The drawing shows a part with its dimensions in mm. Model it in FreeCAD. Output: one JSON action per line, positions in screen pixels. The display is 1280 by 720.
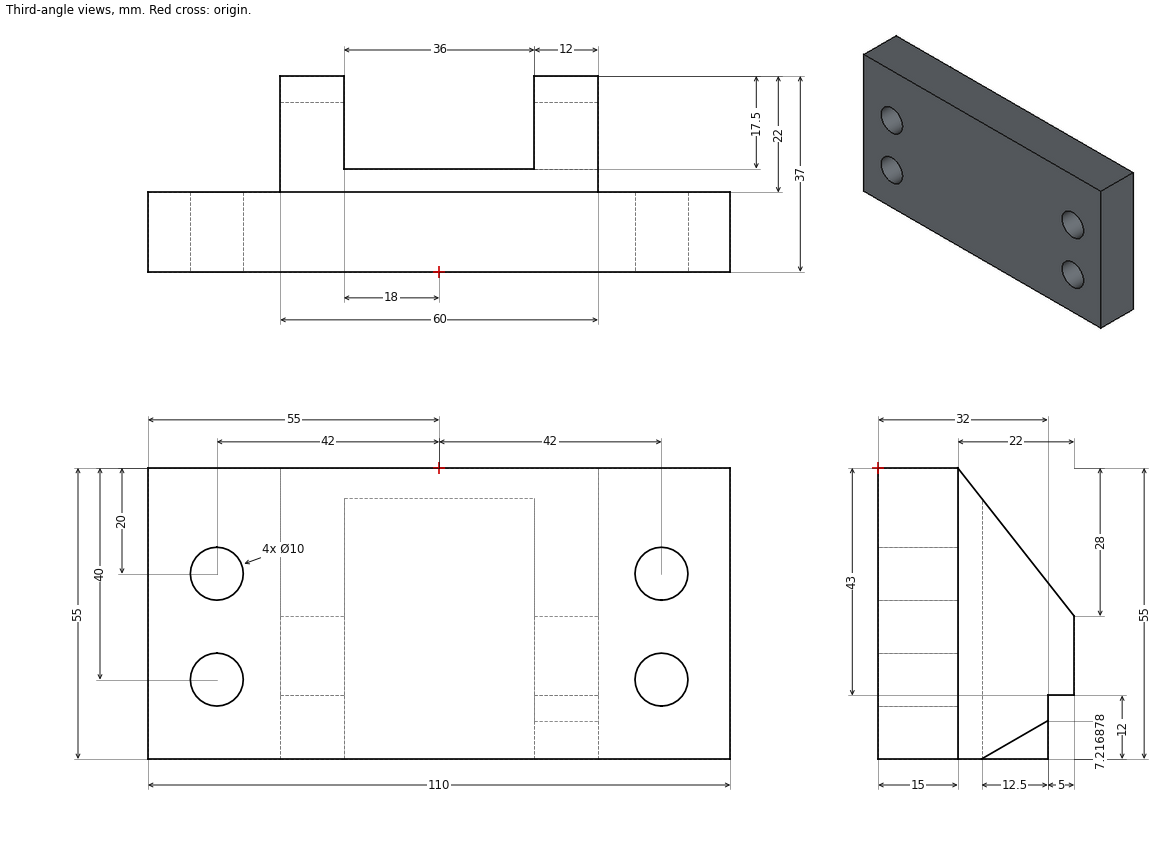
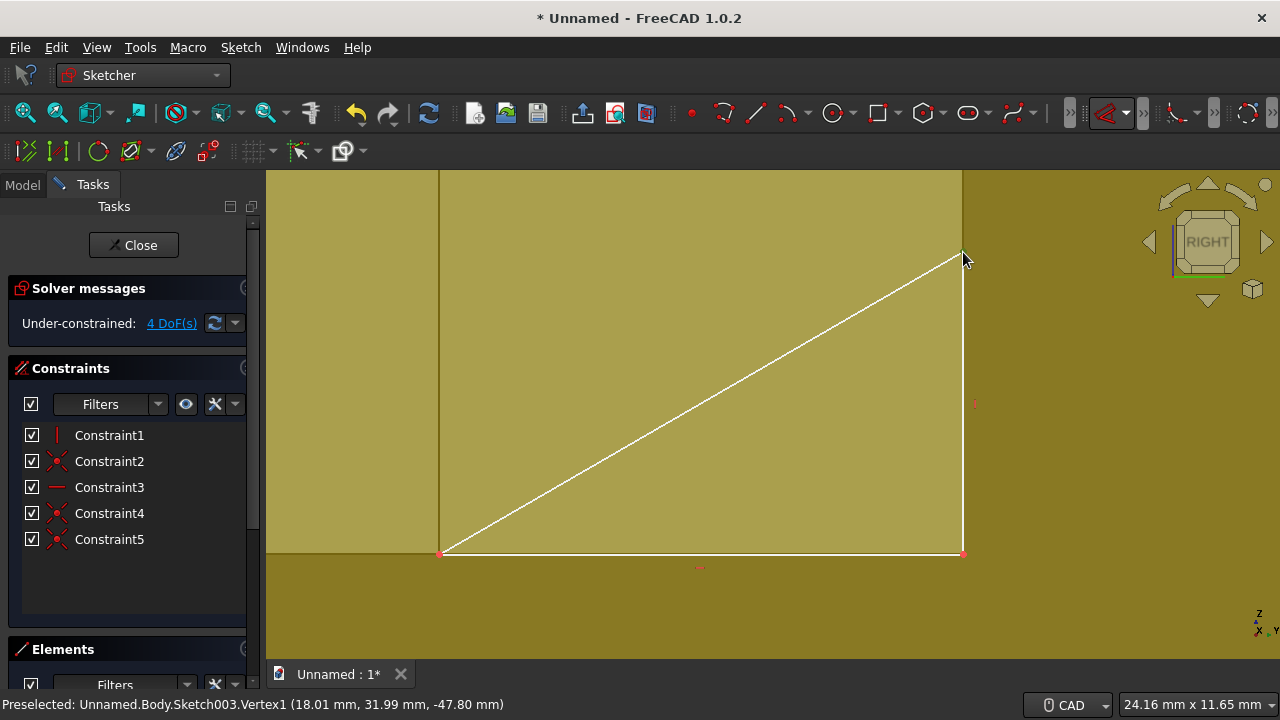
{"action": "key", "text": "l"}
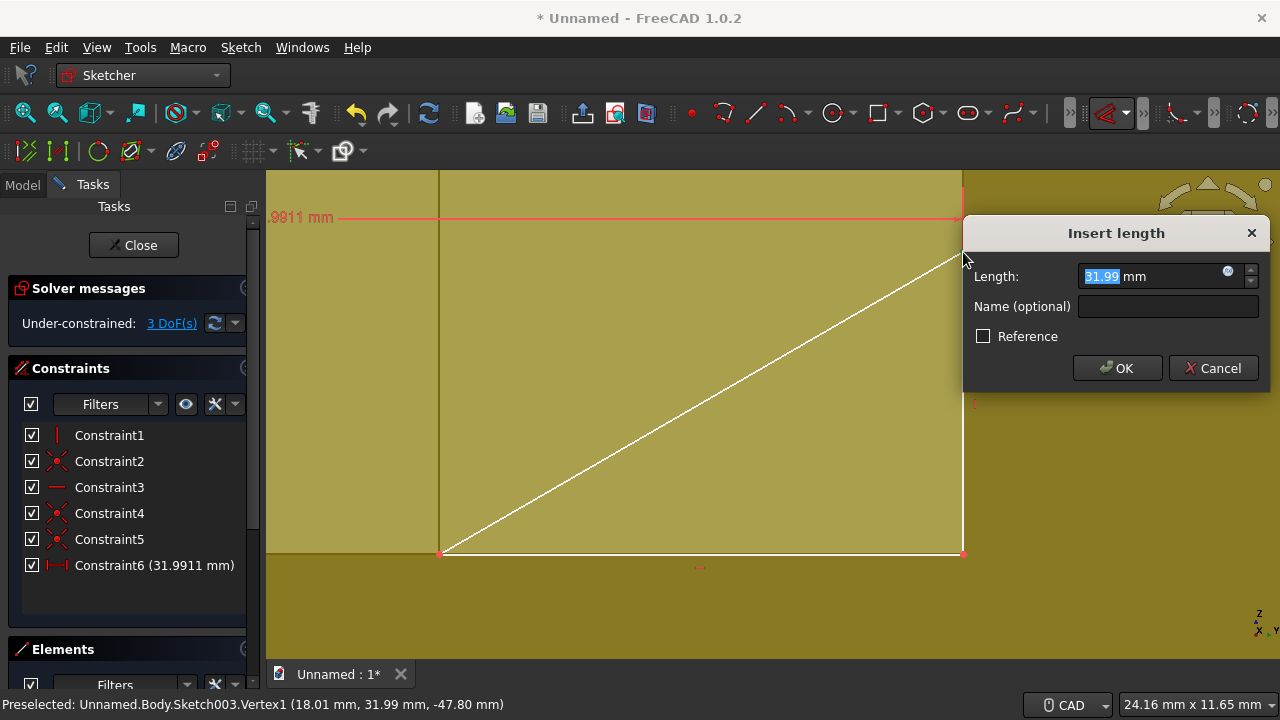
{"action": "type", "text": "32"}
{"action": "key", "text": "Return"}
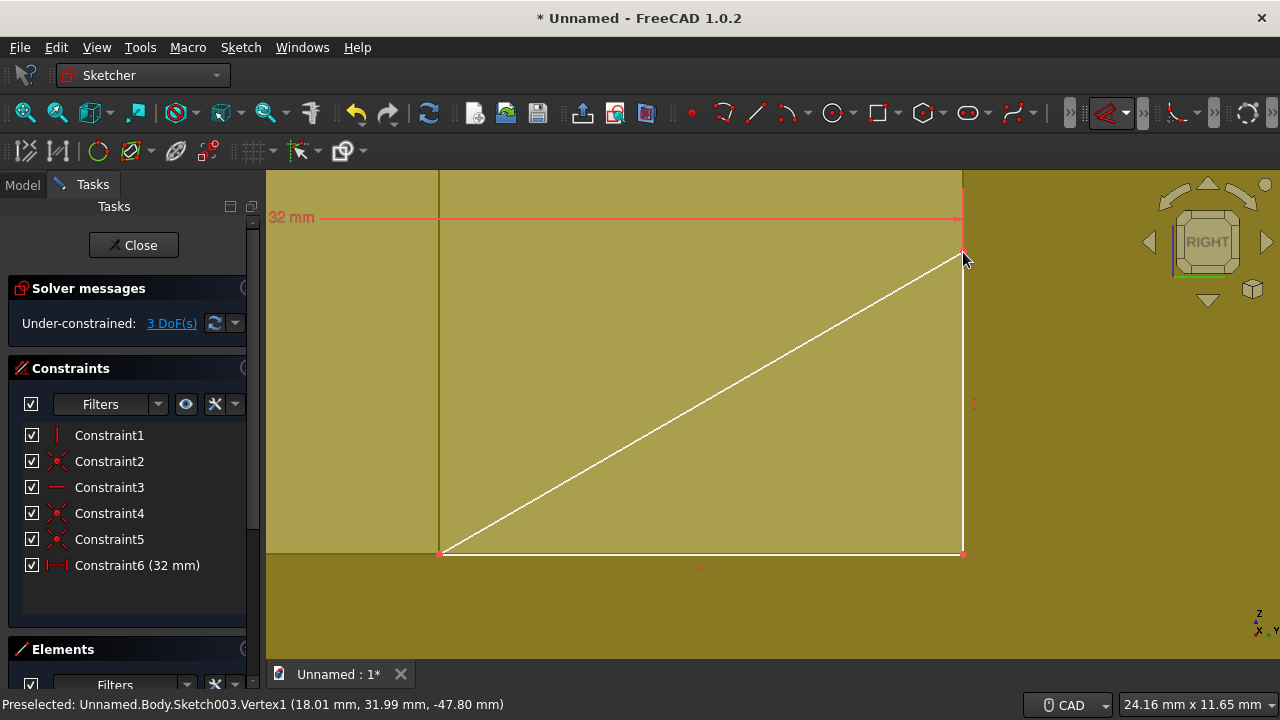
{"action": "left_click", "coordinate": [963, 555]}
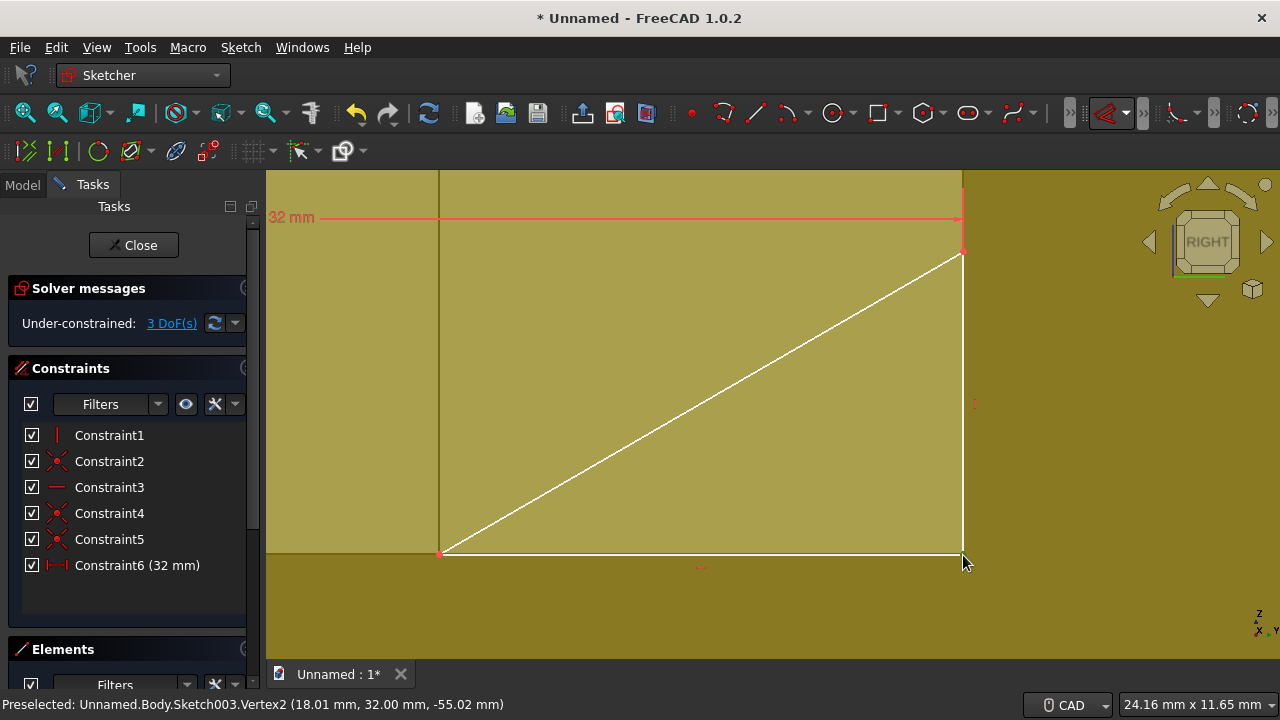
{"action": "key", "text": "i"}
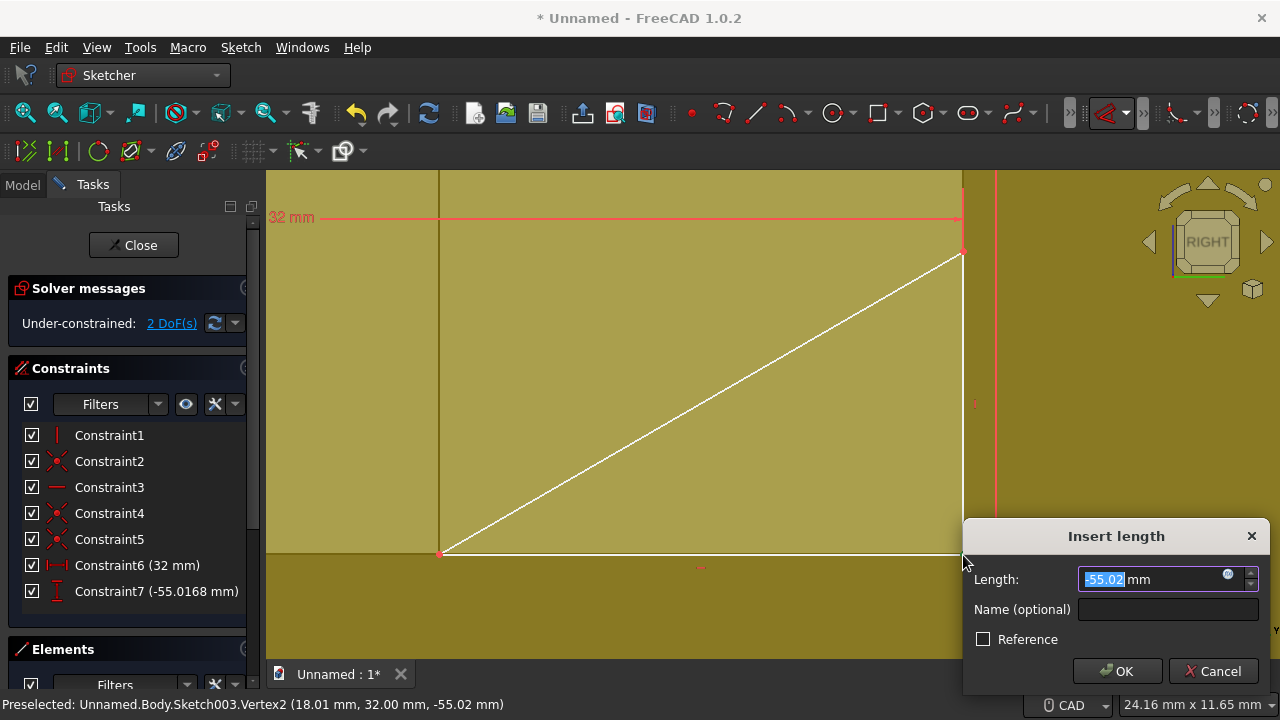
{"action": "type", "text": "-55"}
{"action": "key", "text": "Return"}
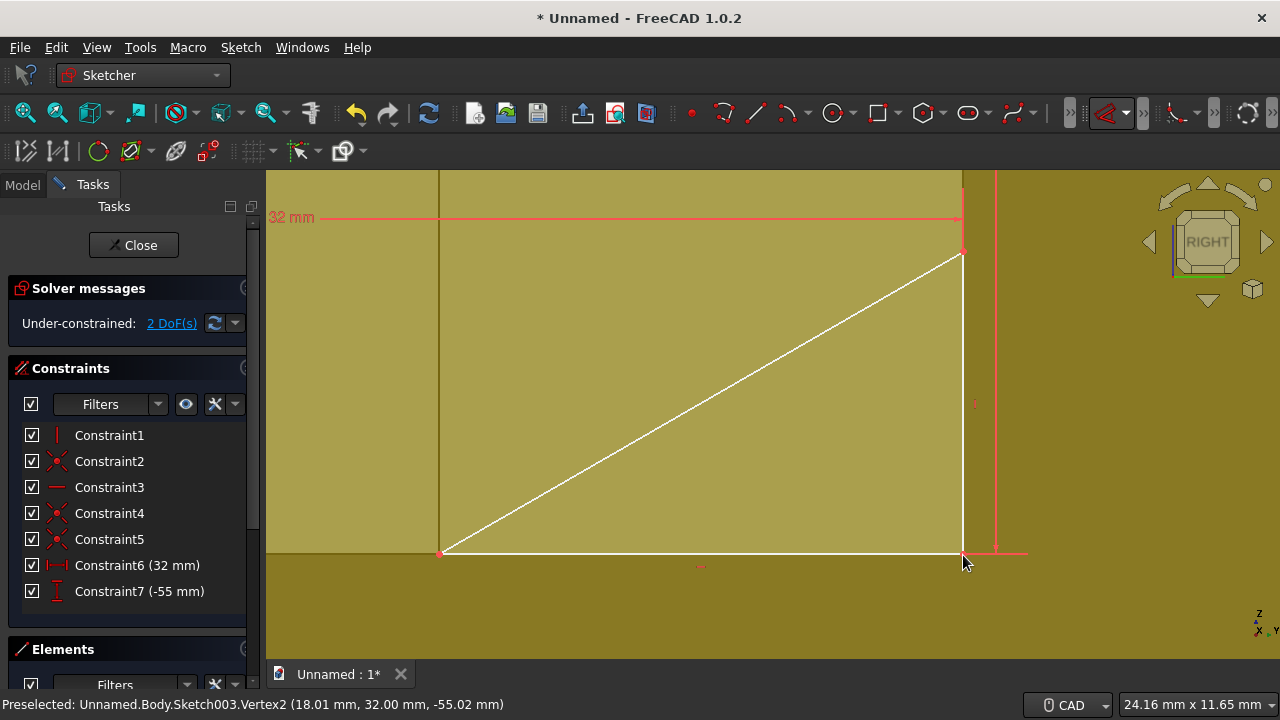
{"action": "left_click", "coordinate": [806, 554]}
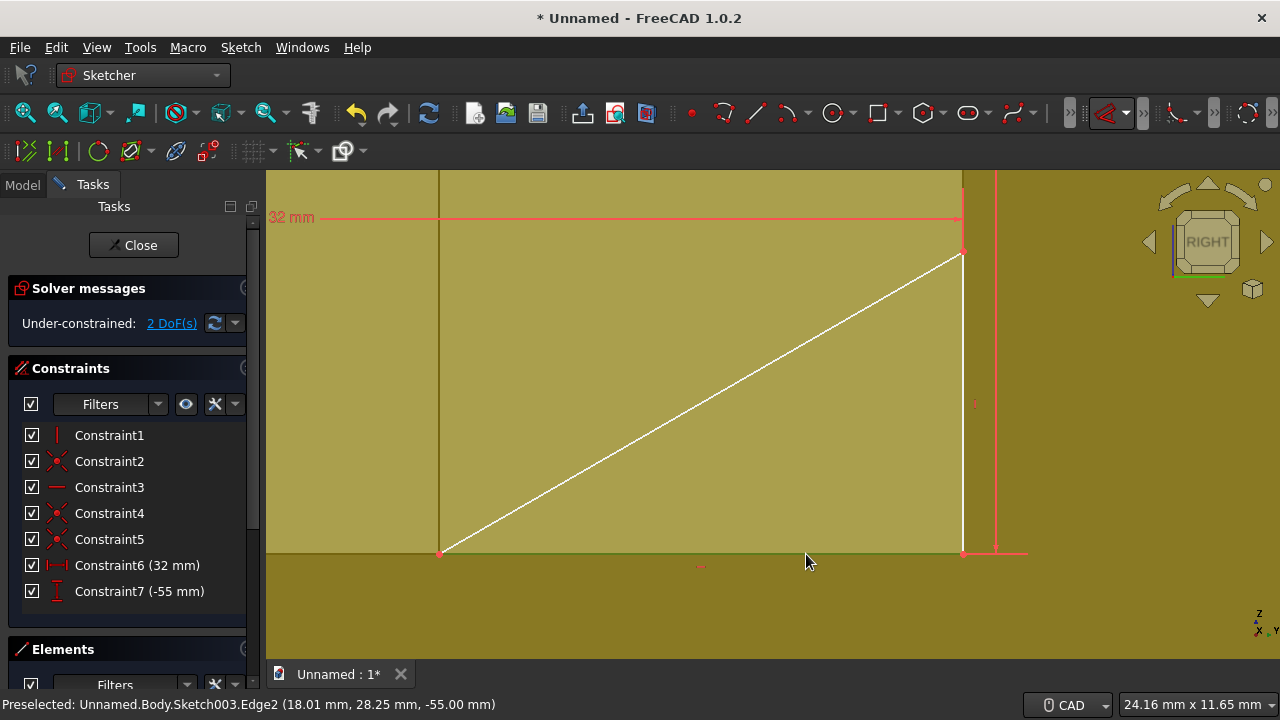
{"action": "left_click", "coordinate": [1128, 114]}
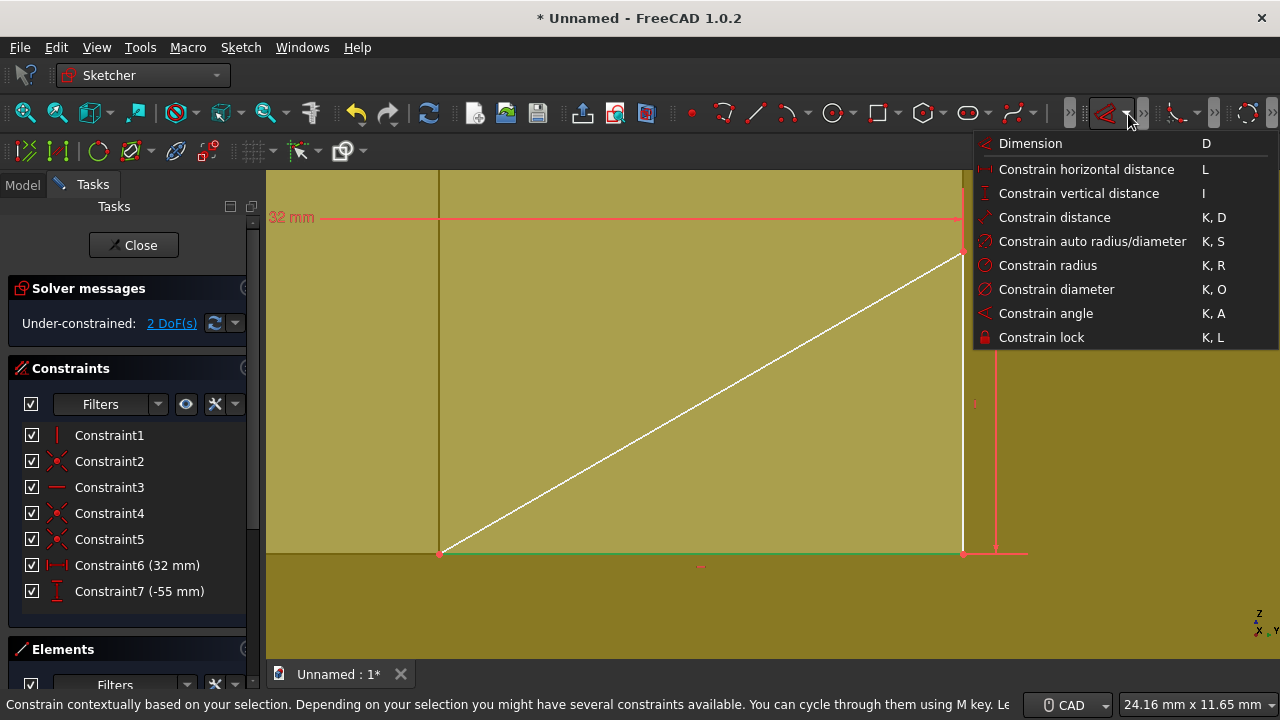
{"action": "left_click", "coordinate": [1126, 169]}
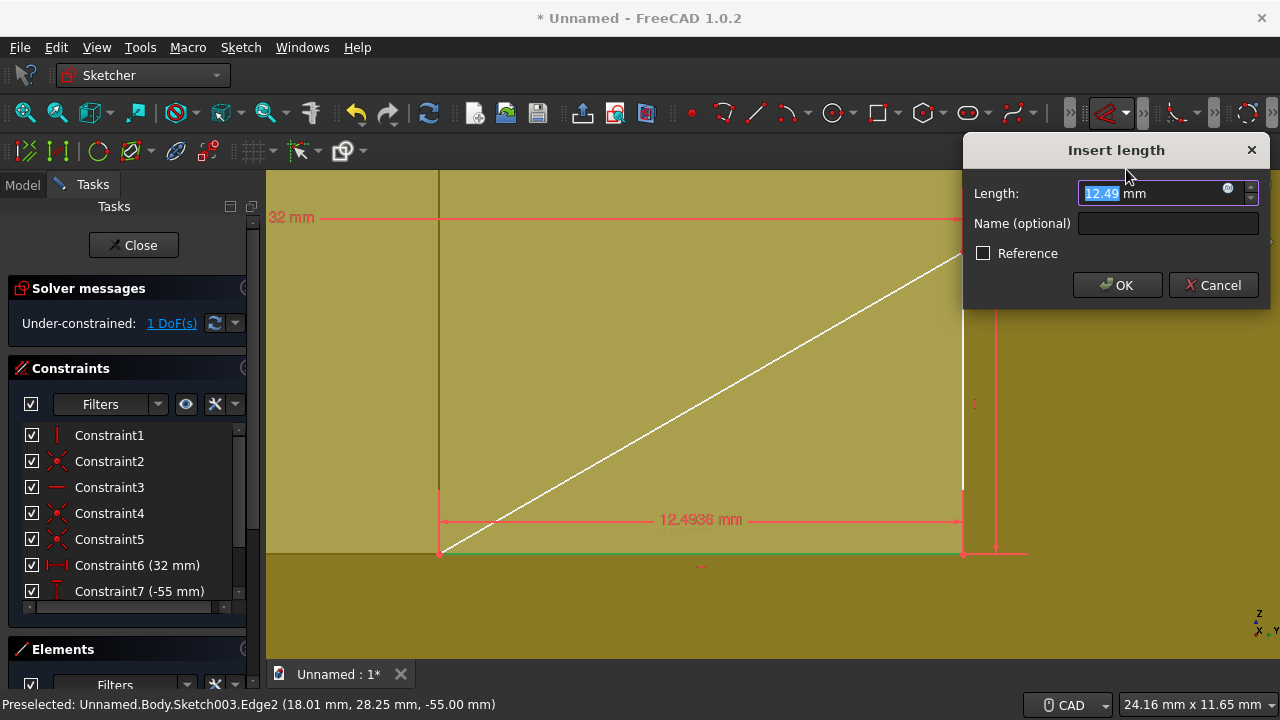
{"action": "type", "text": "12.5"}
{"action": "key", "text": "Return"}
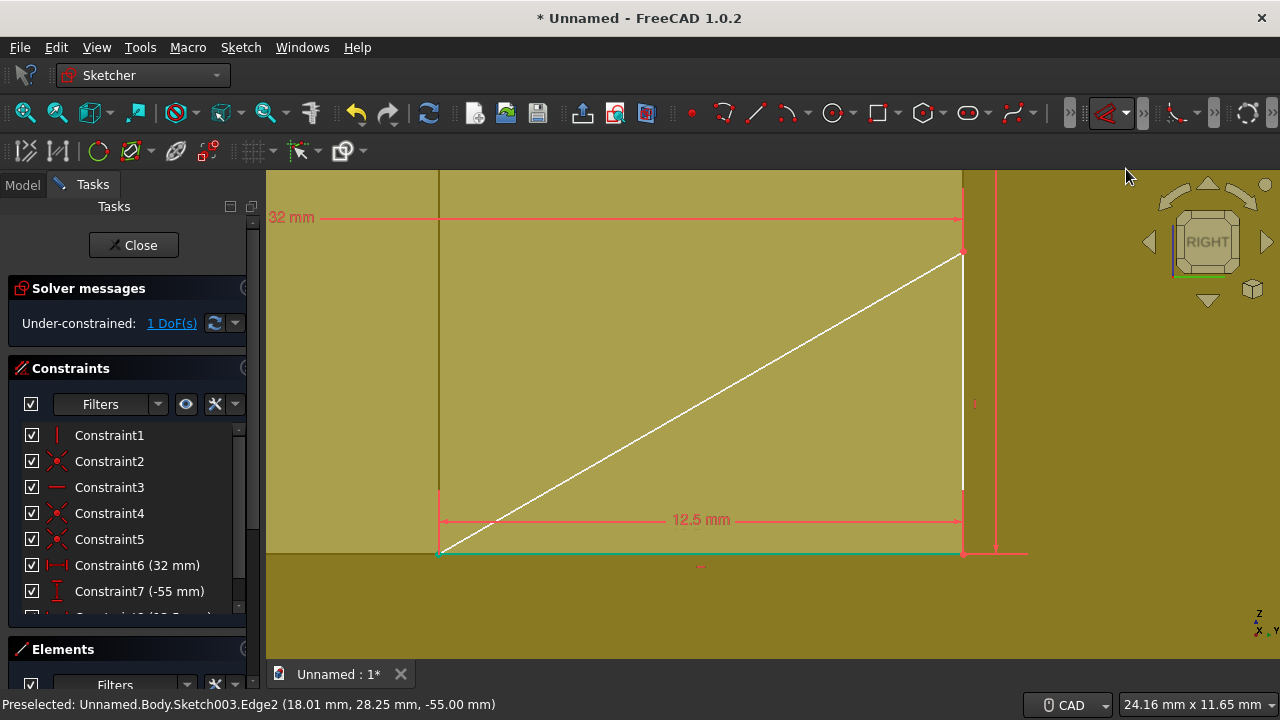
{"action": "left_click", "coordinate": [963, 343]}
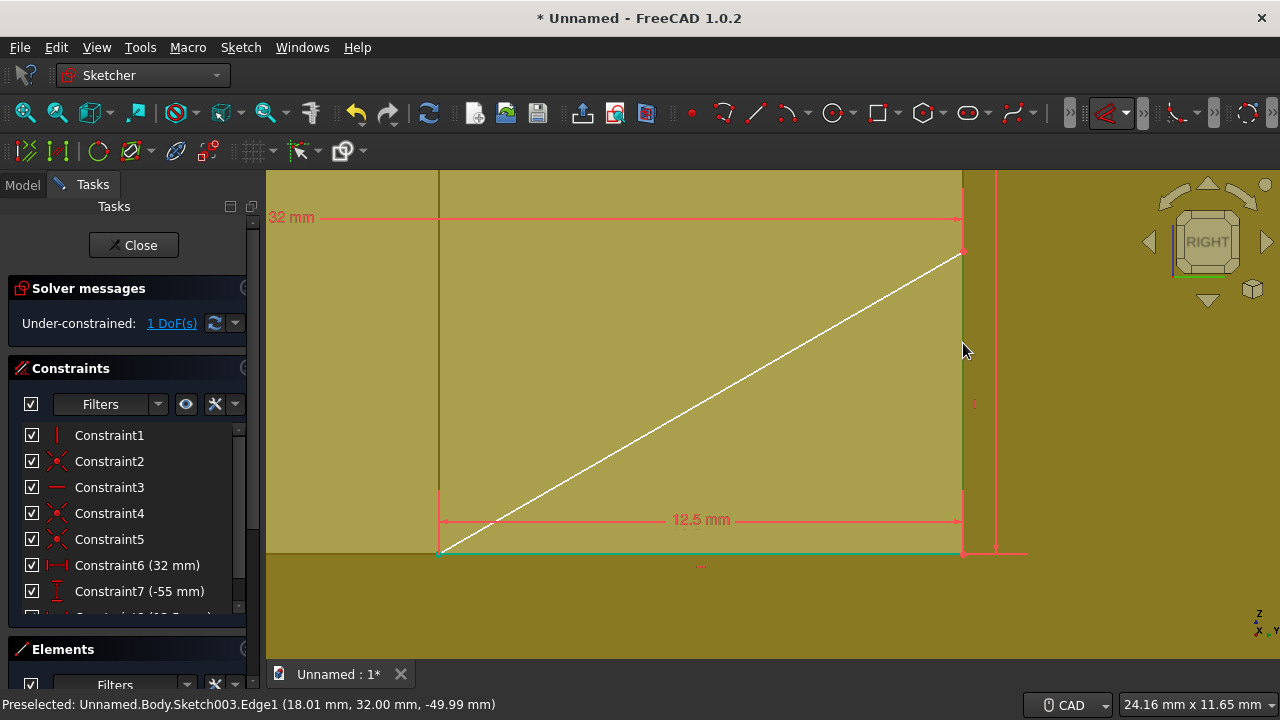
{"action": "key", "text": "i"}